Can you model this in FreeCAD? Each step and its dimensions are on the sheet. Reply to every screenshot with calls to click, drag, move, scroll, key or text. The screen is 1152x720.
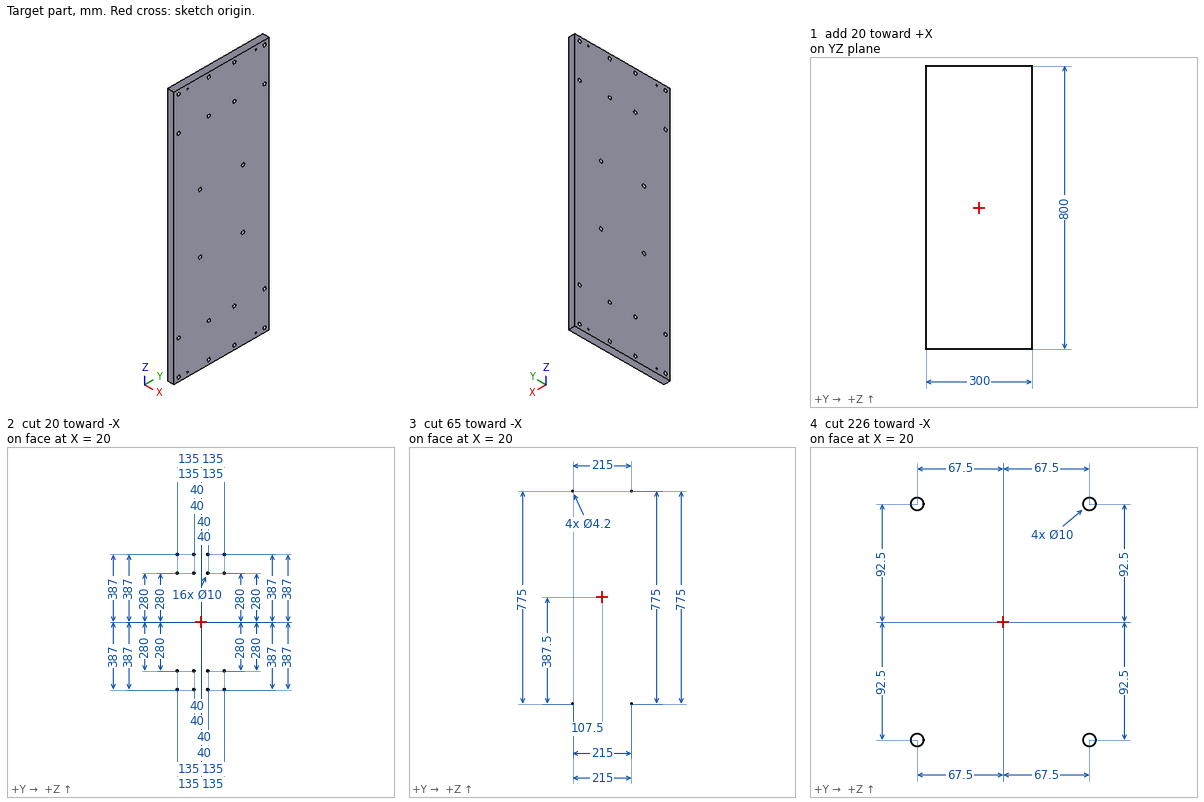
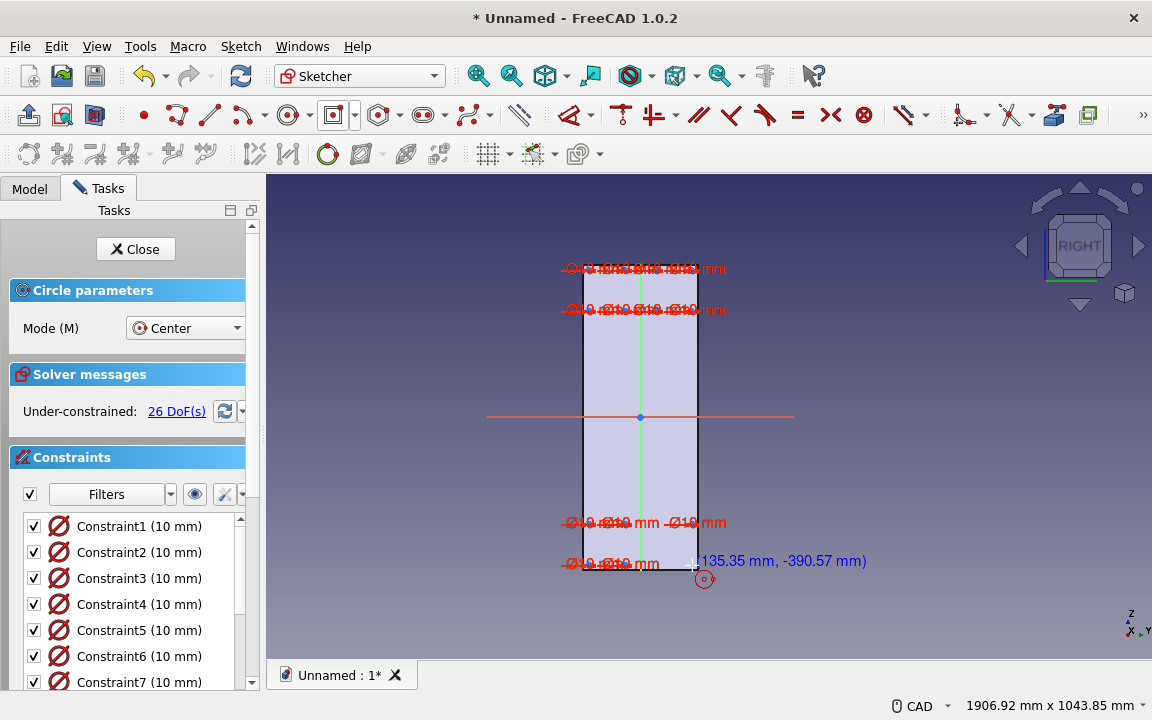
click(692, 565)
move(693, 563)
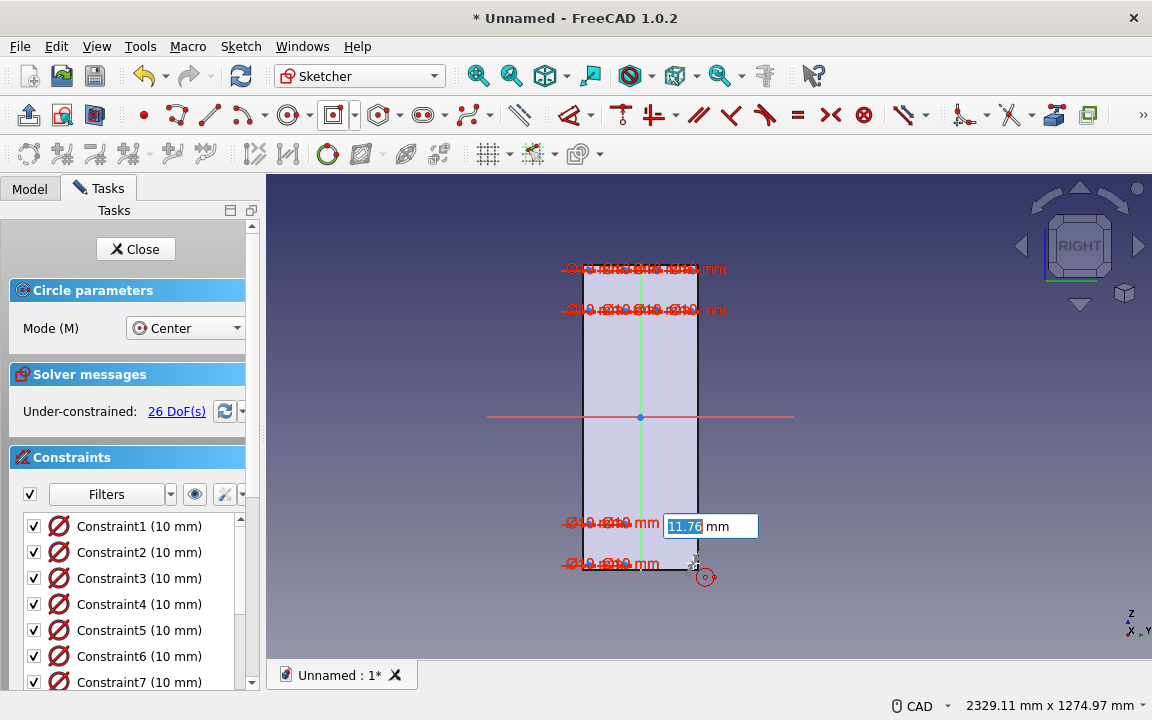
text(10)
key(Return)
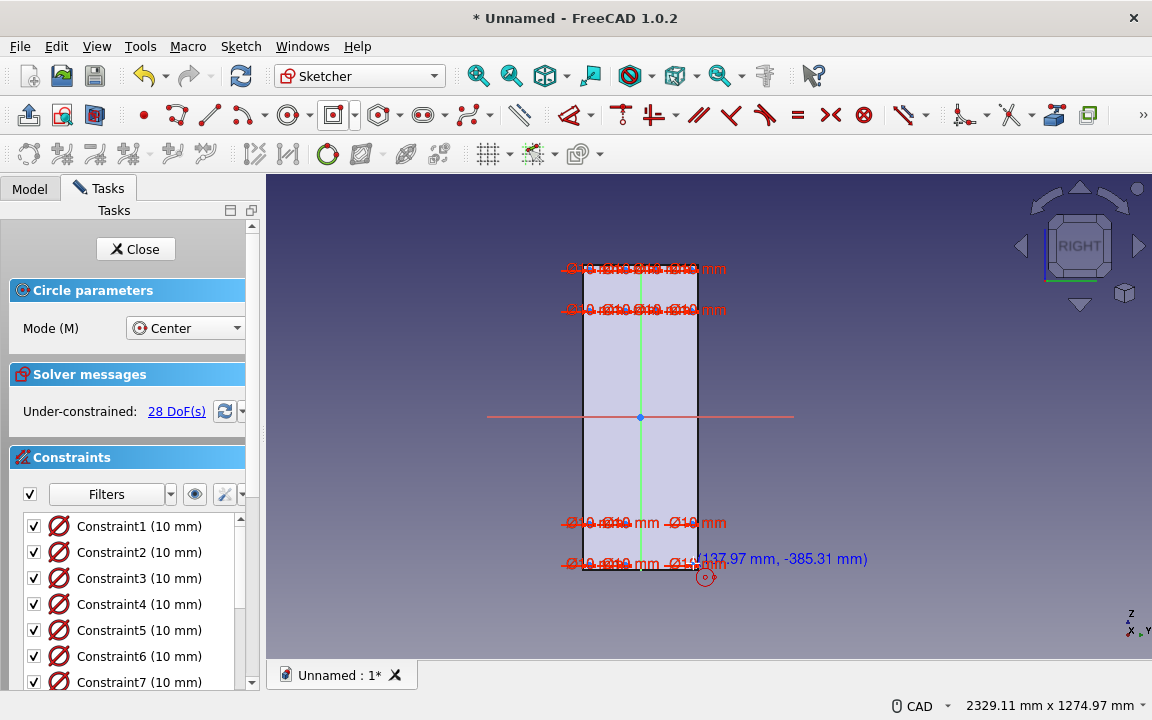
scroll(656, 565, up, 13)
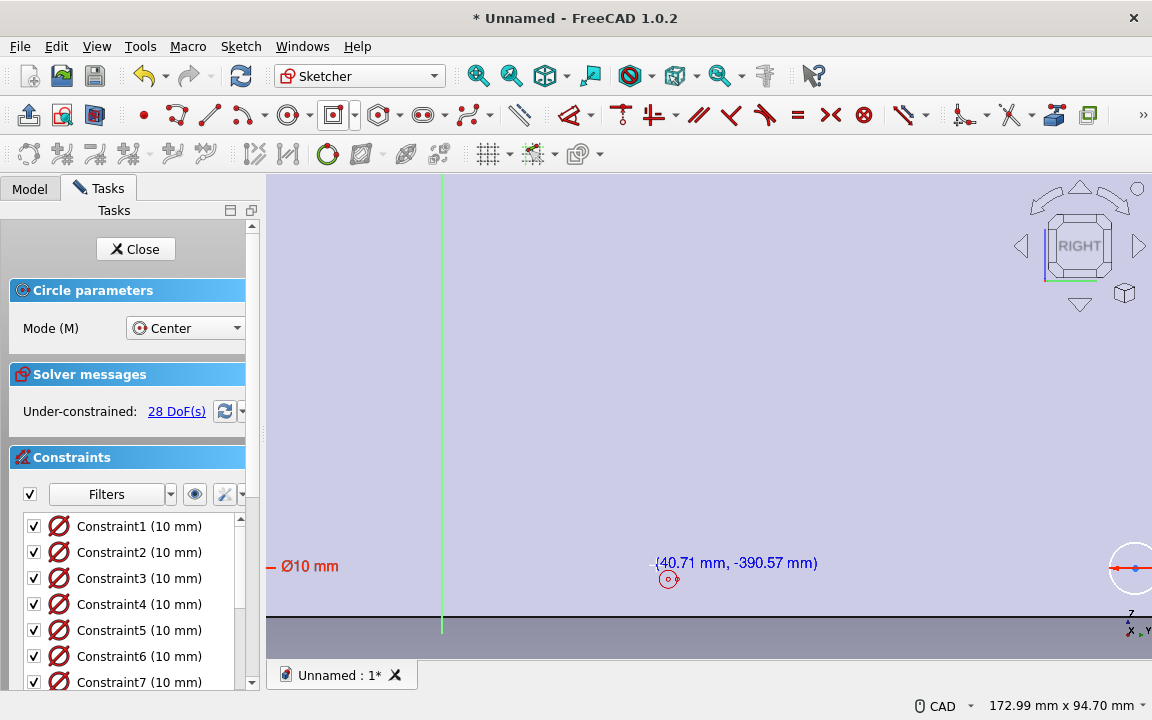
scroll(656, 565, down, 13)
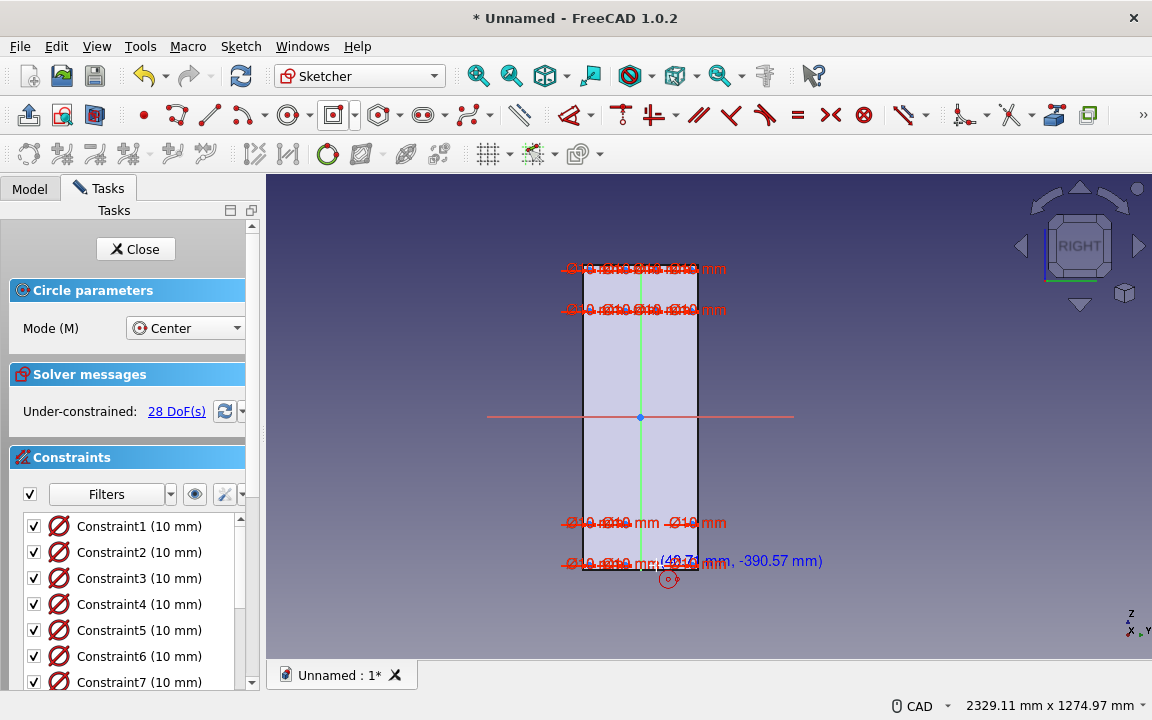
click(656, 565)
move(657, 563)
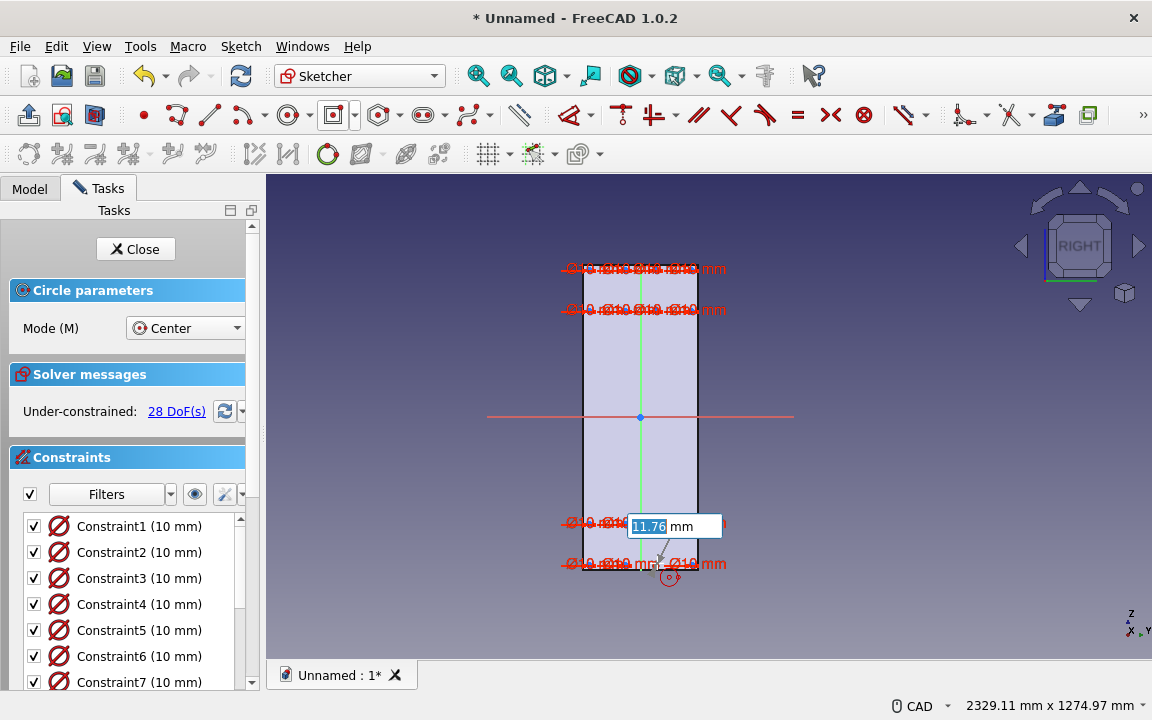
text(10)
key(Return)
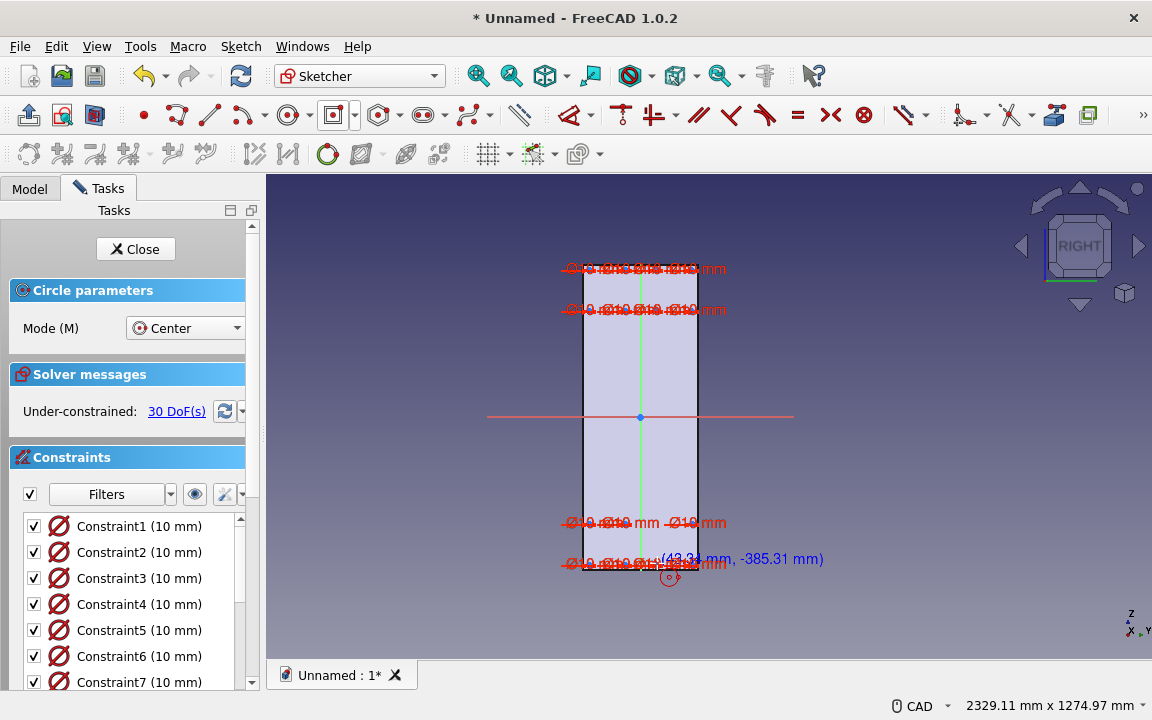
scroll(656, 524, up, 13)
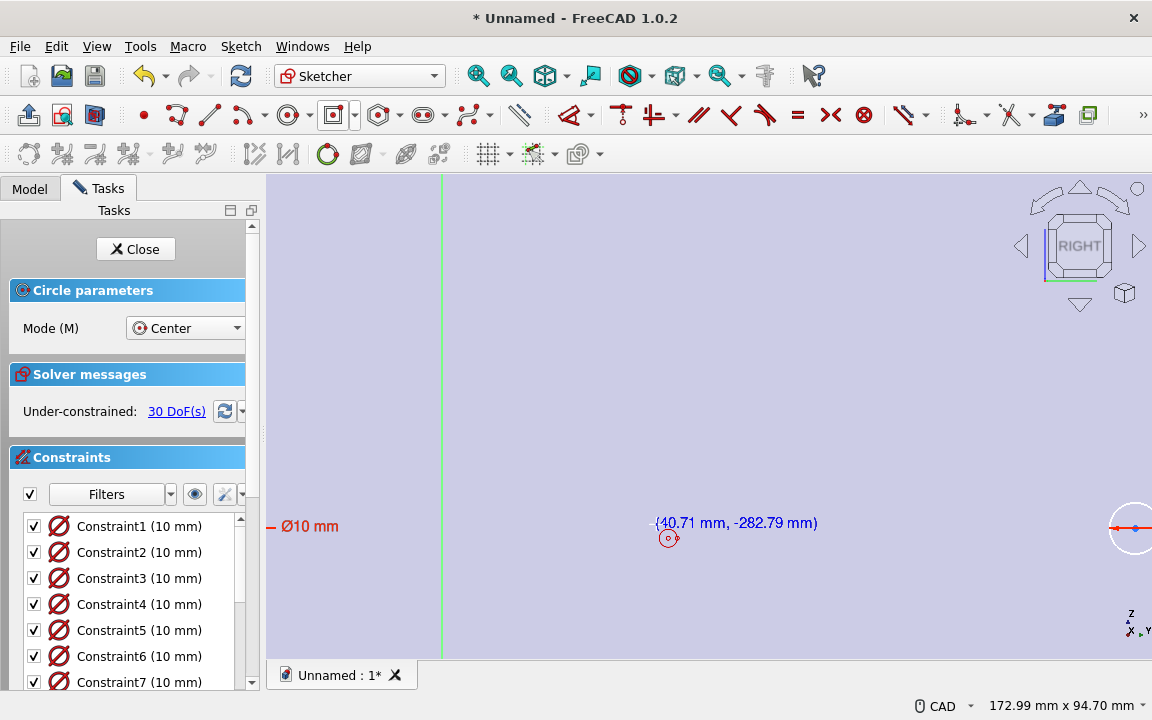
scroll(656, 524, down, 13)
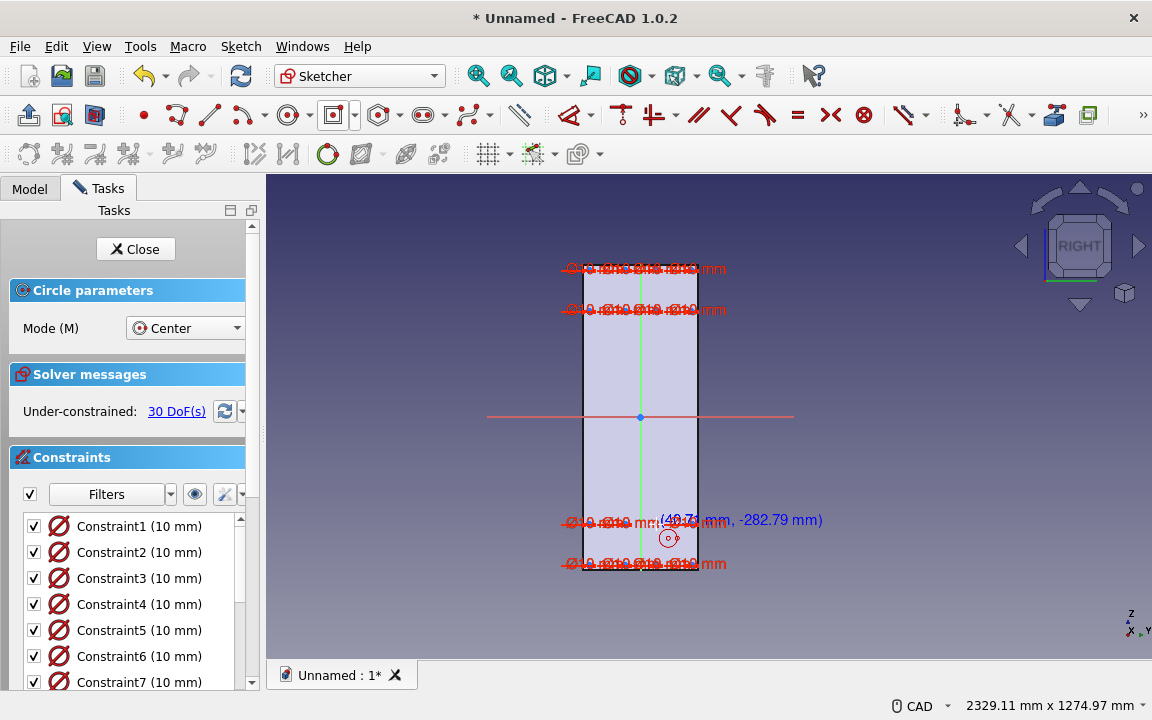
click(656, 524)
move(657, 523)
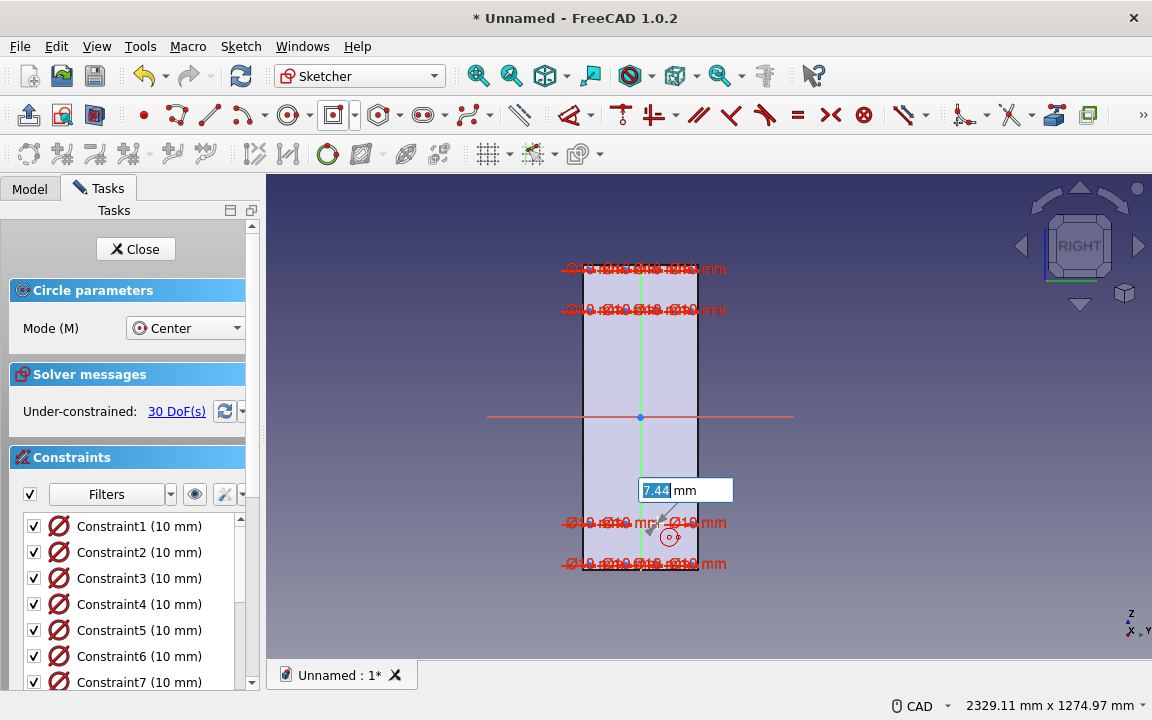
text(10)
key(Return)
key(Escape)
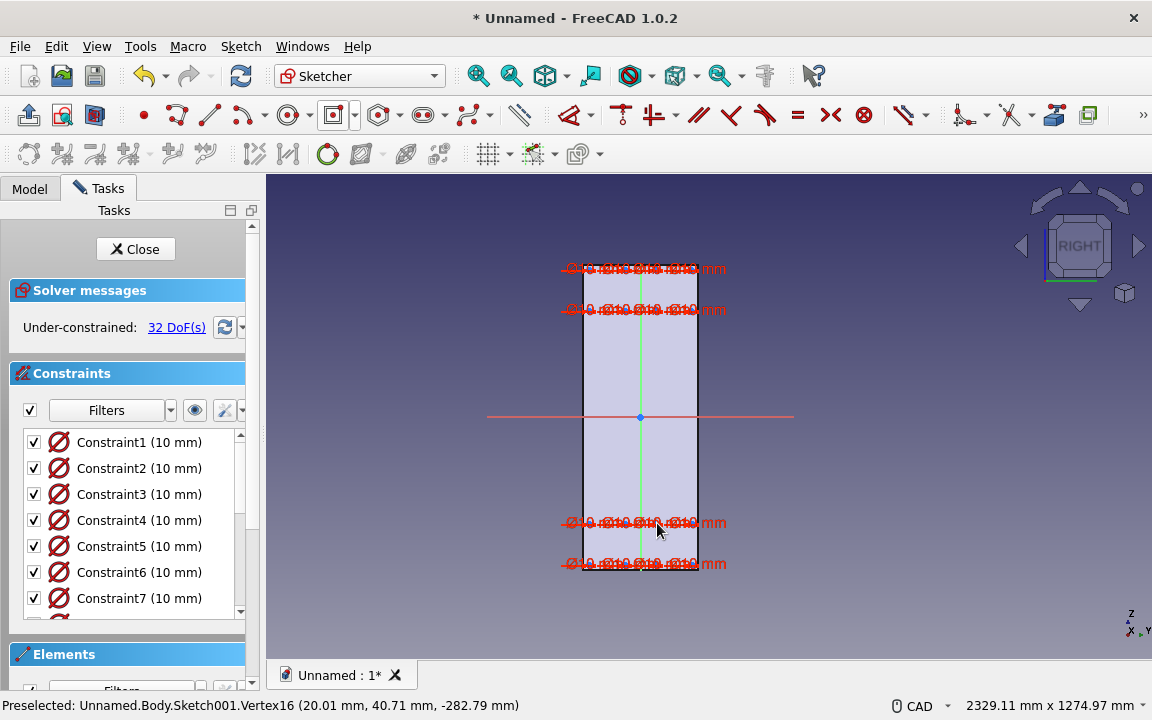
scroll(656, 312, up, 5)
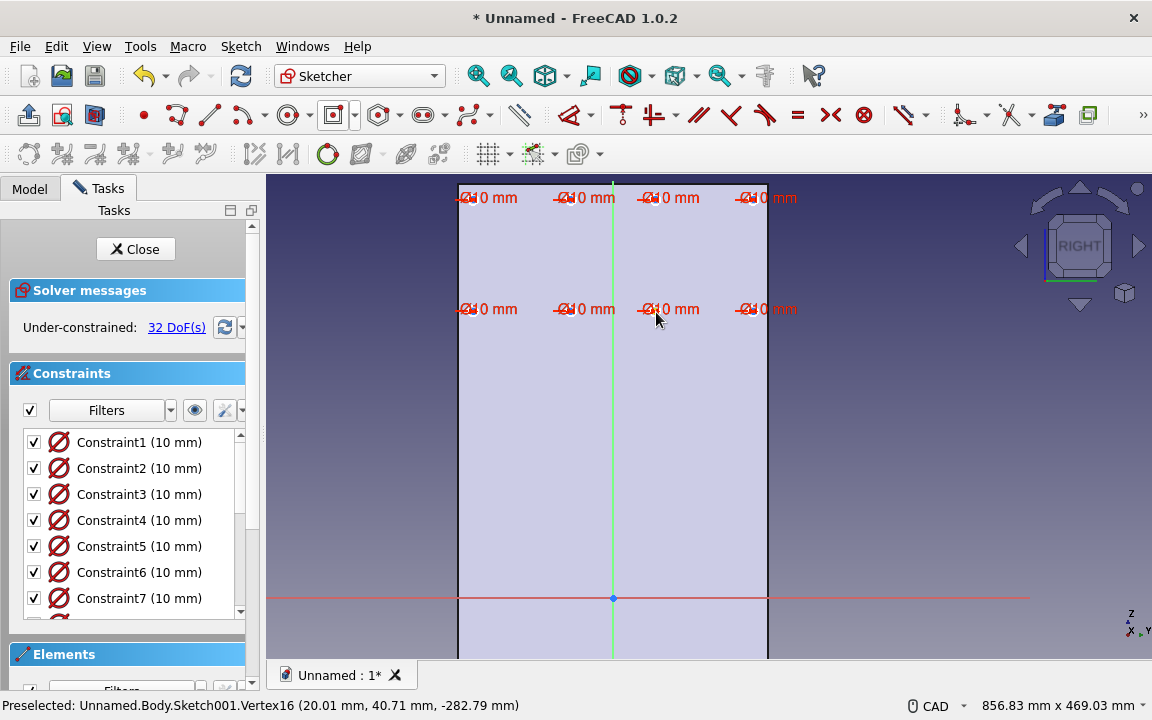
click(655, 311)